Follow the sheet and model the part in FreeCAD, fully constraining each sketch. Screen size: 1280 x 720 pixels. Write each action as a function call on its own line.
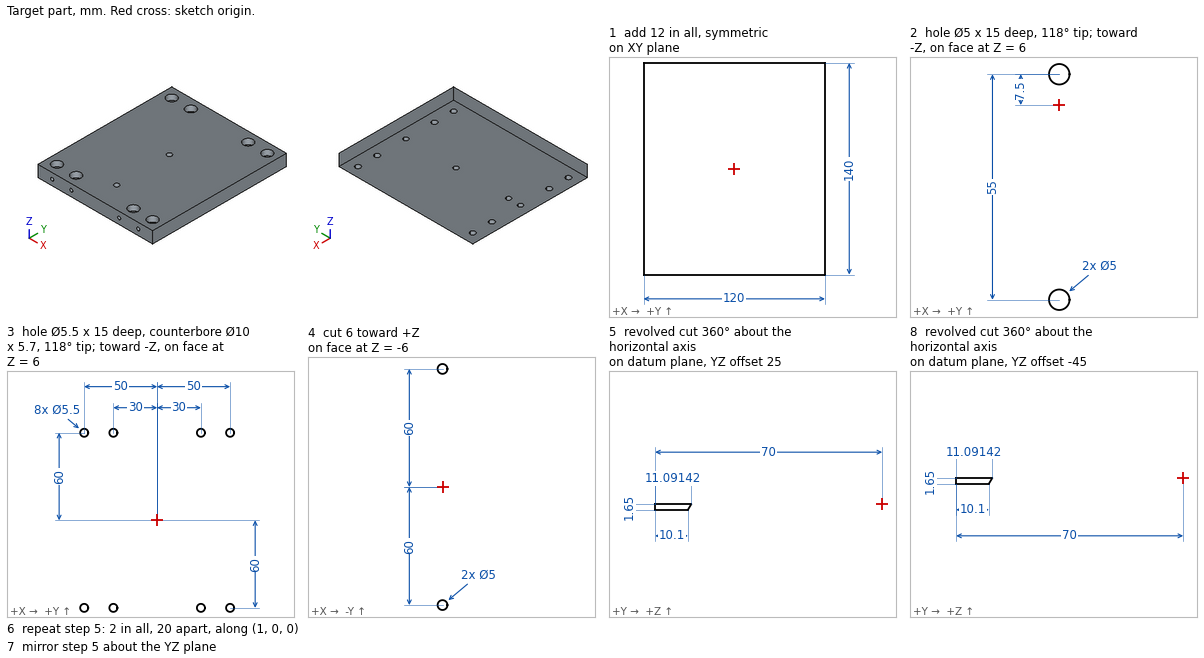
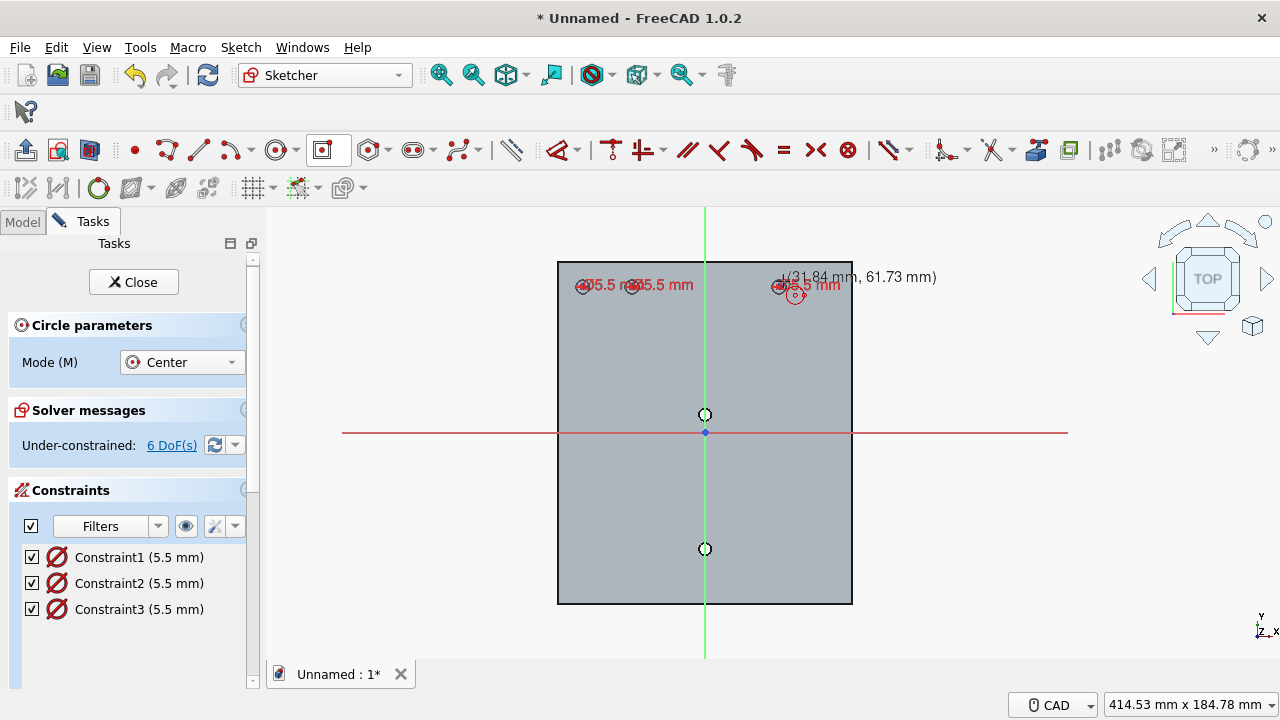
scroll(827, 286, up, 7)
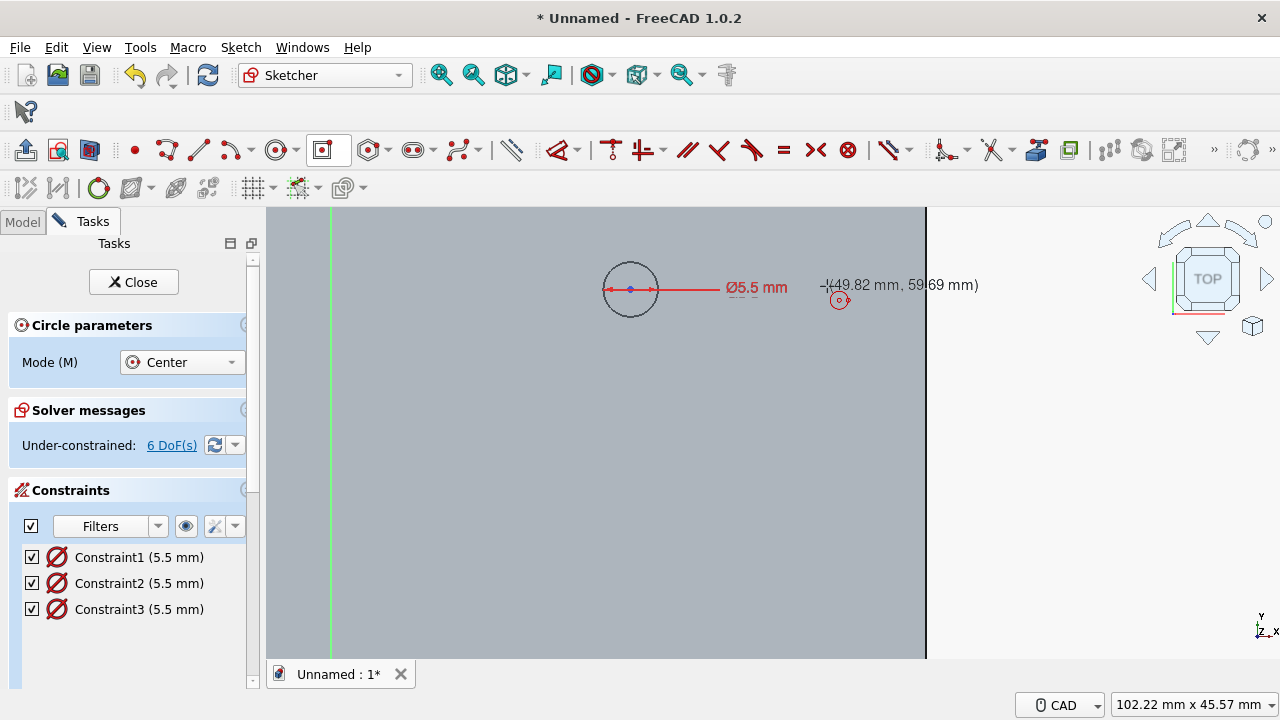
scroll(827, 286, down, 7)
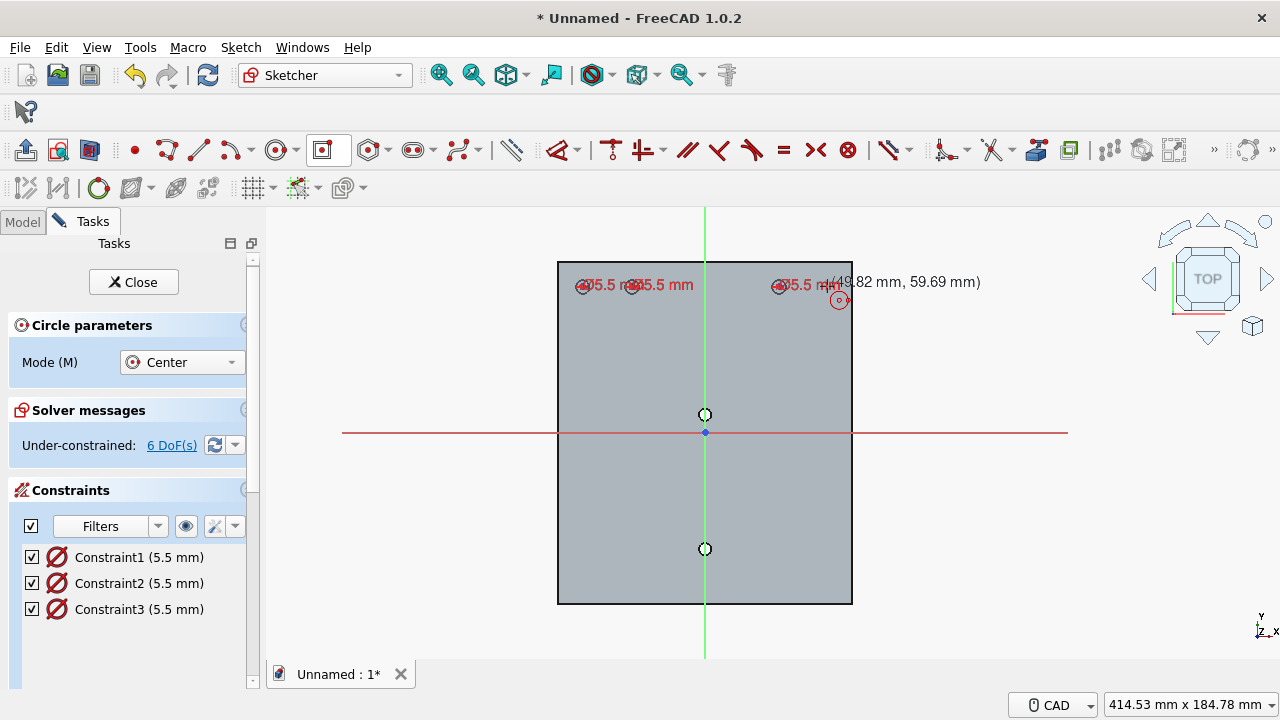
click(827, 286)
move(832, 281)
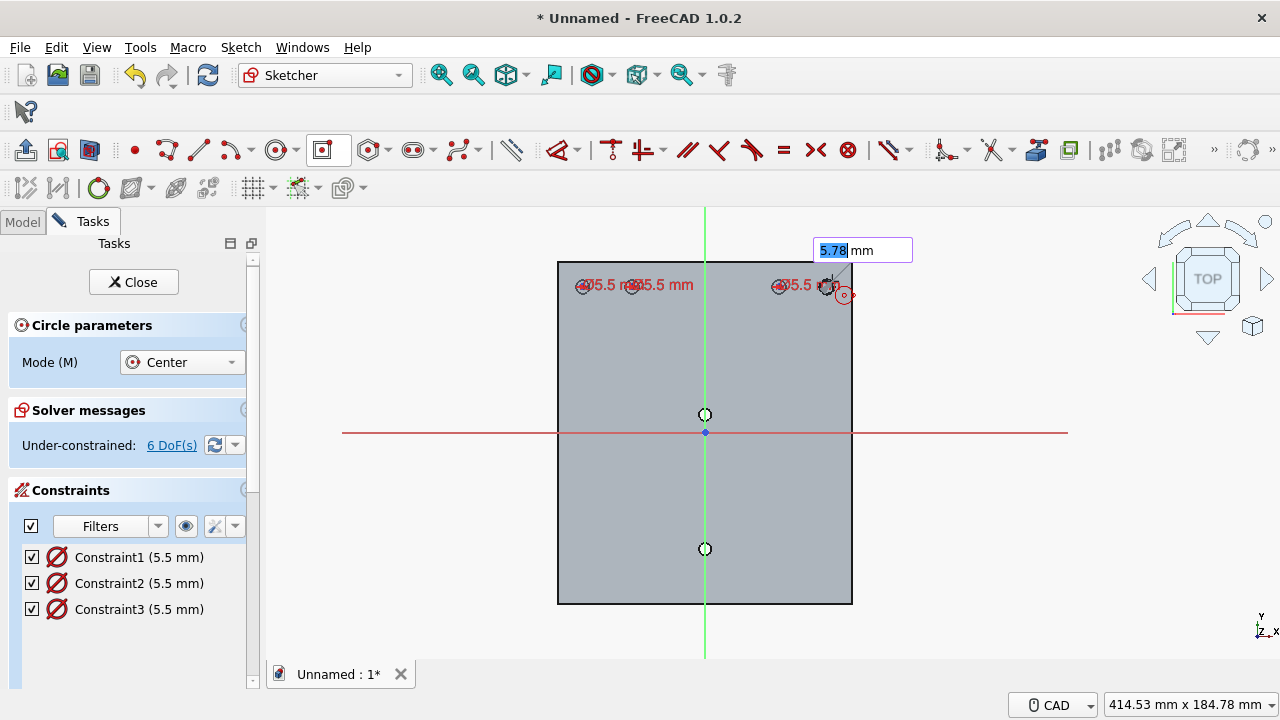
text(5.5)
key(Return)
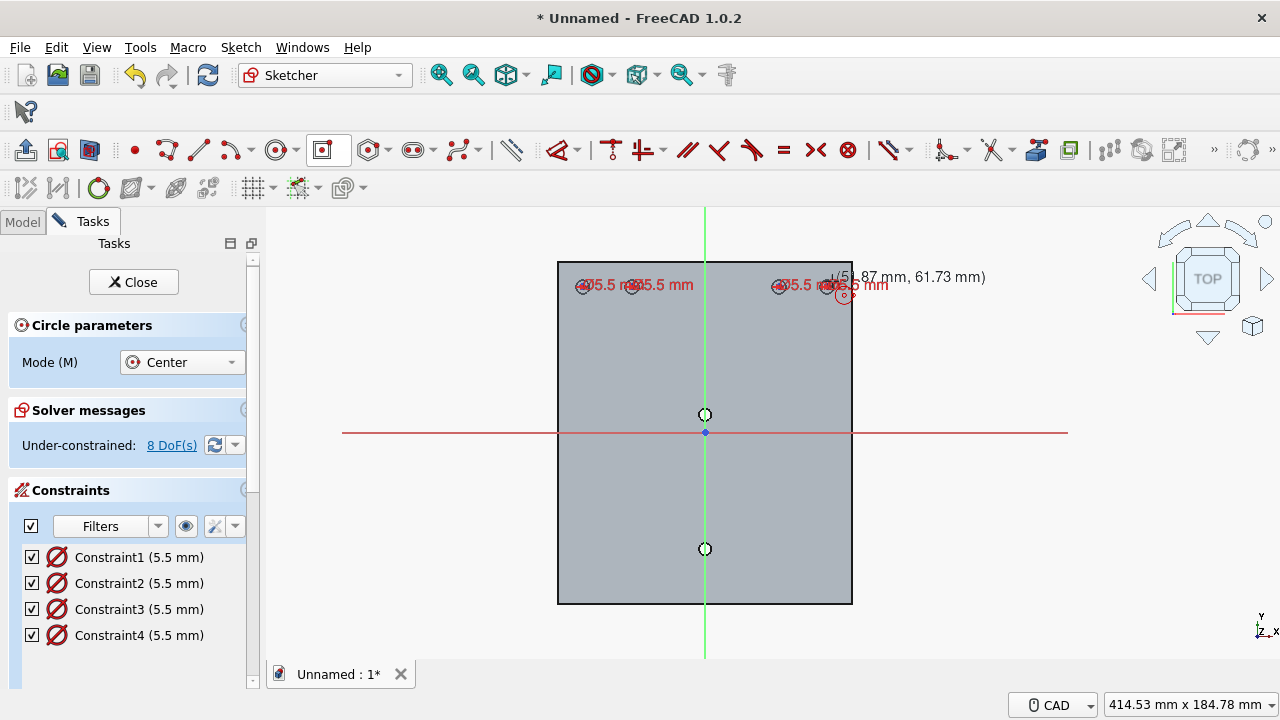
scroll(827, 580, up, 7)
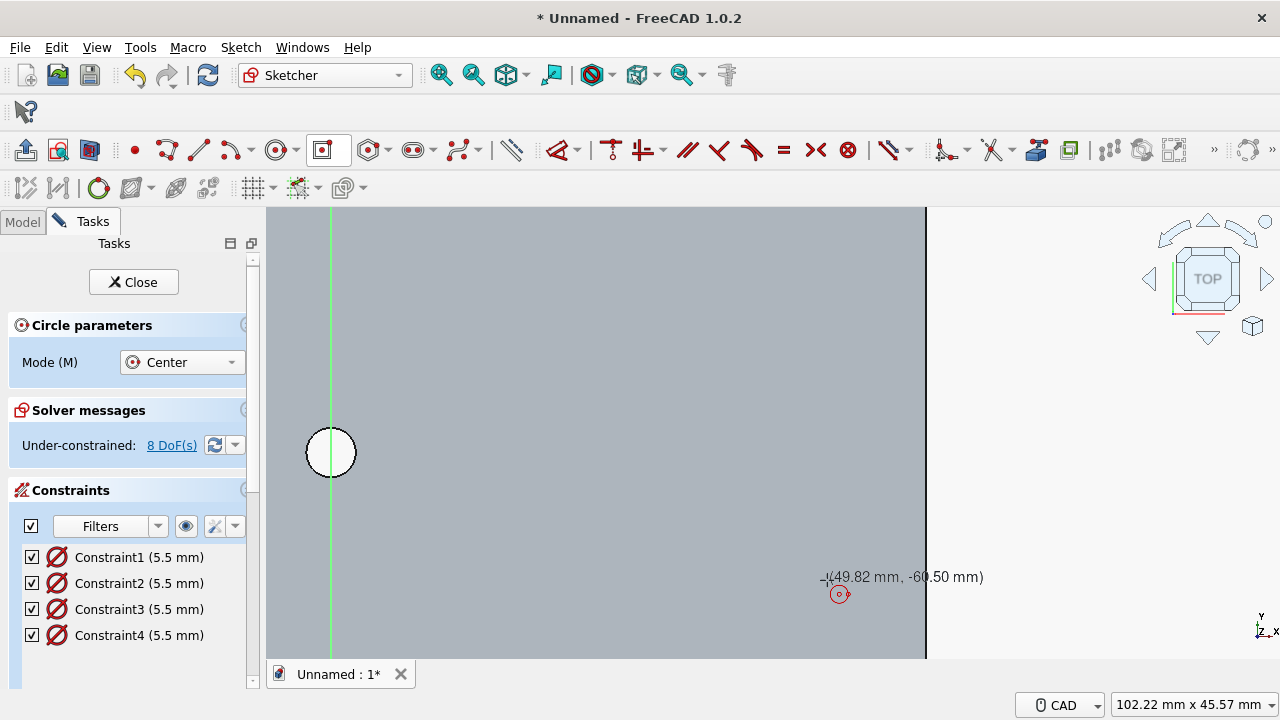
scroll(827, 581, down, 7)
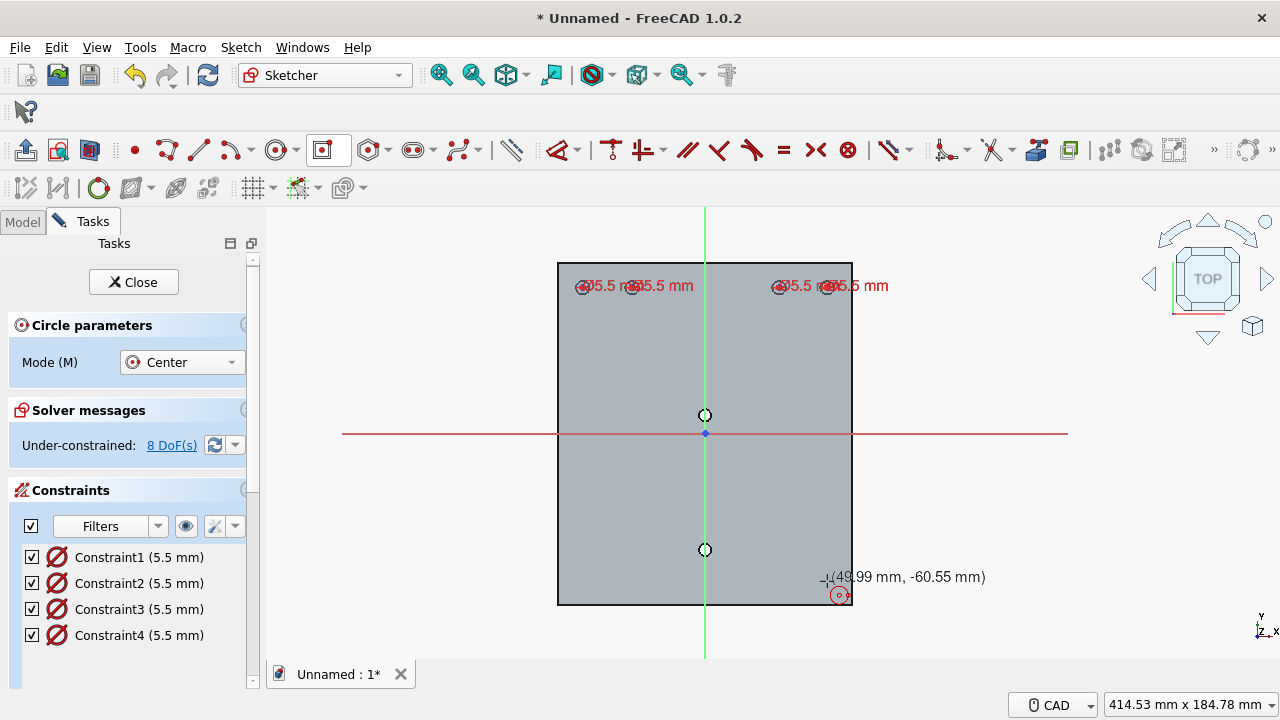
click(827, 581)
move(832, 576)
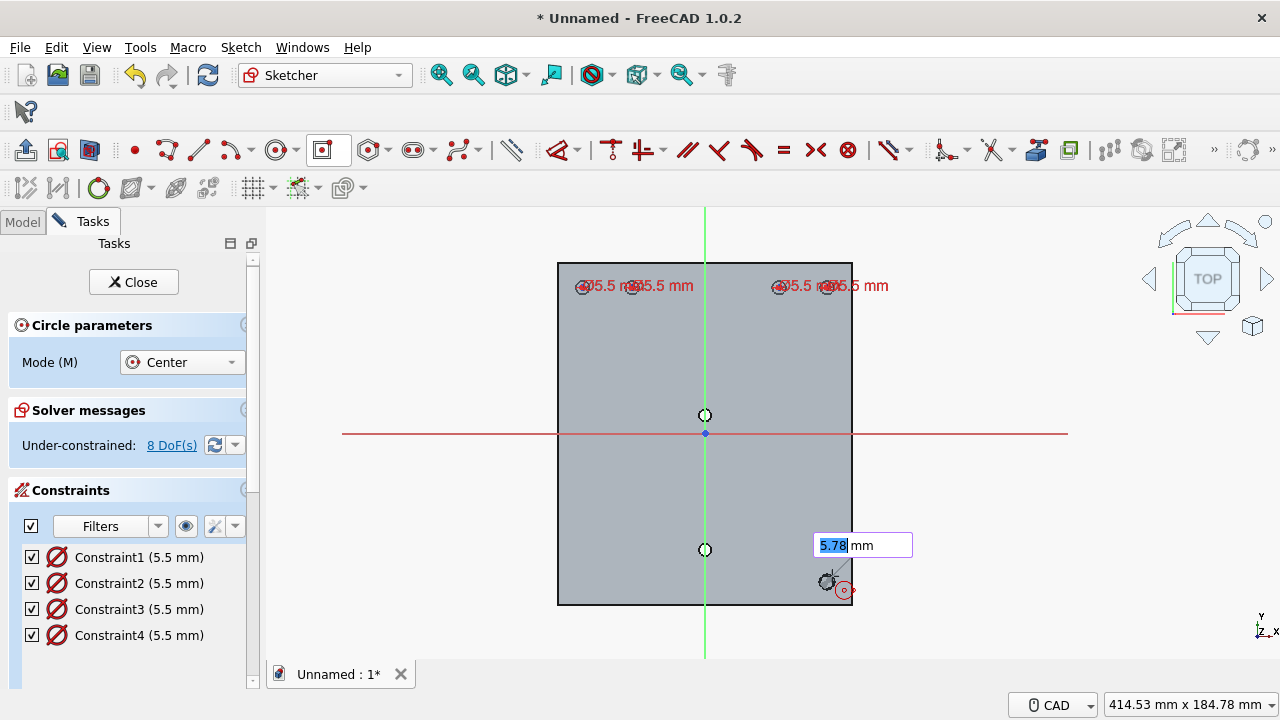
text(5.5)
key(Return)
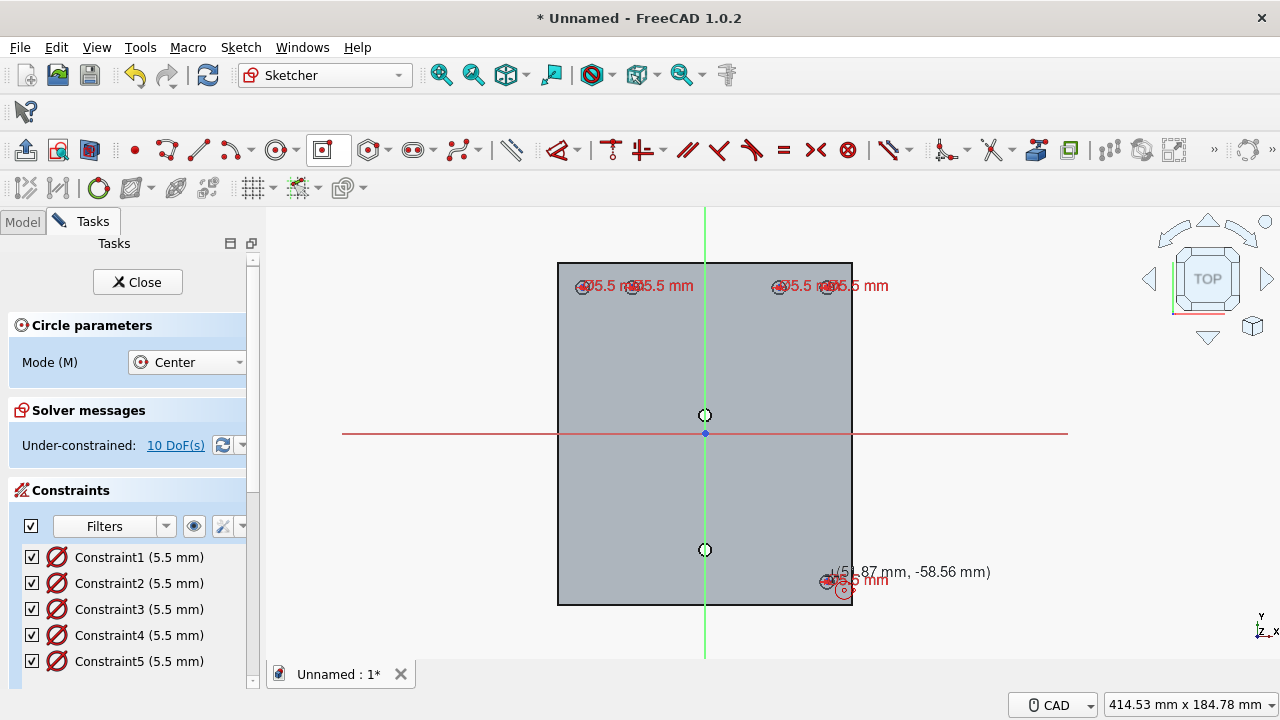
scroll(779, 581, up, 7)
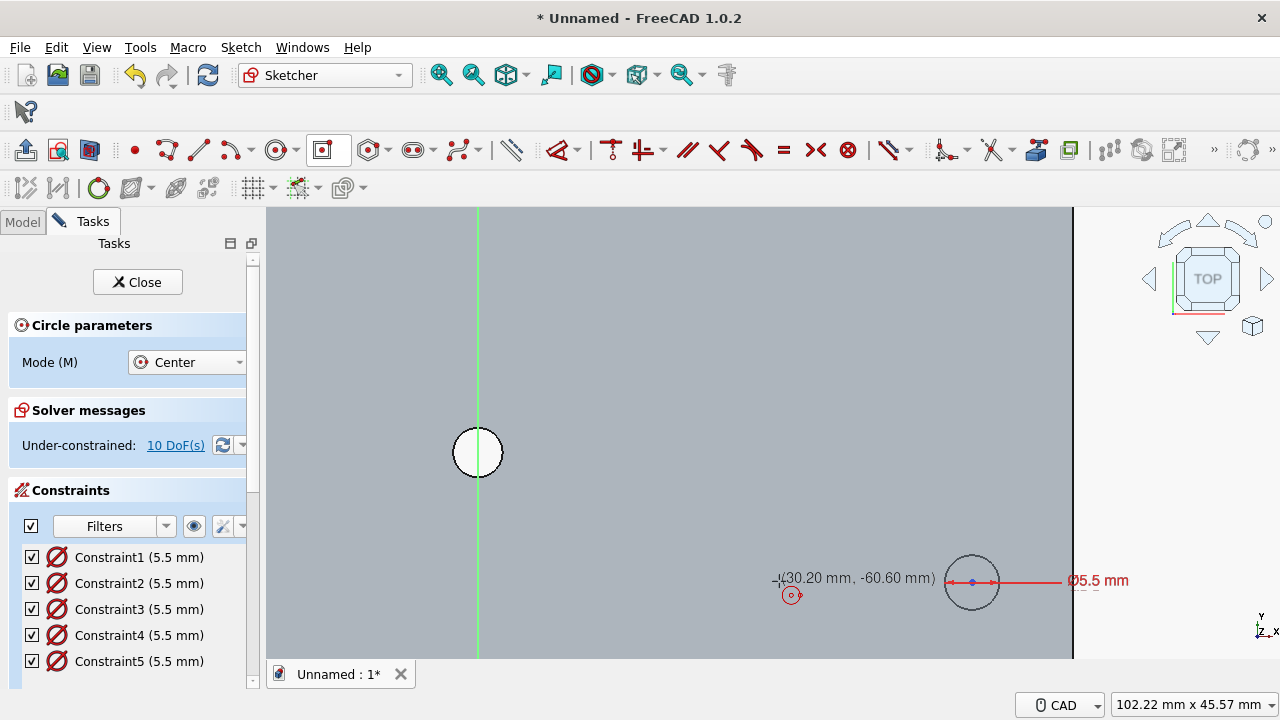
scroll(779, 581, down, 7)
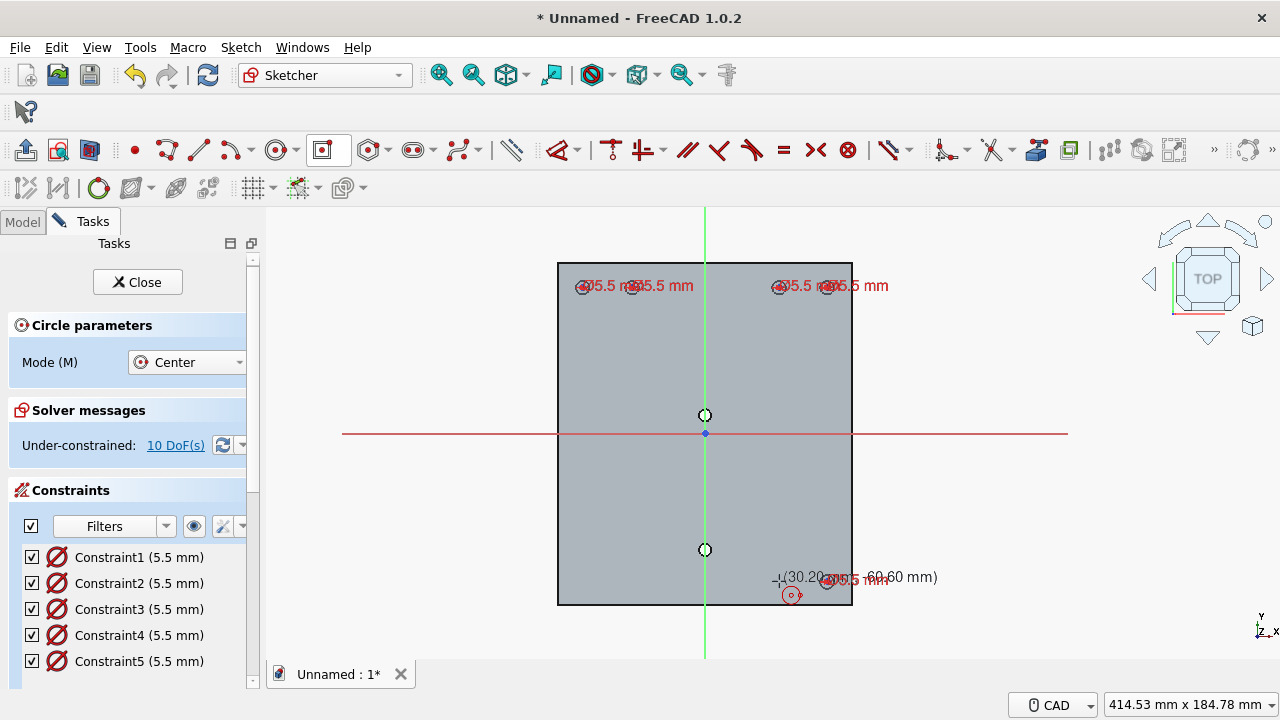
click(779, 581)
move(783, 576)